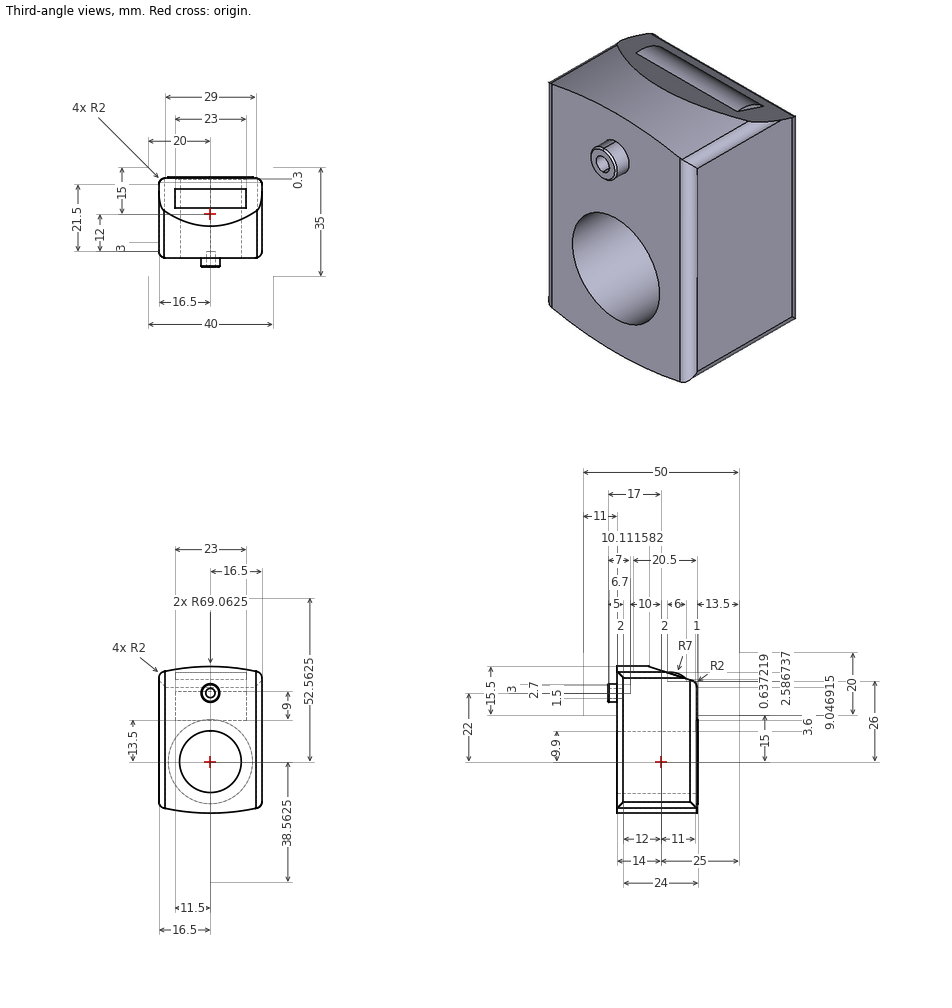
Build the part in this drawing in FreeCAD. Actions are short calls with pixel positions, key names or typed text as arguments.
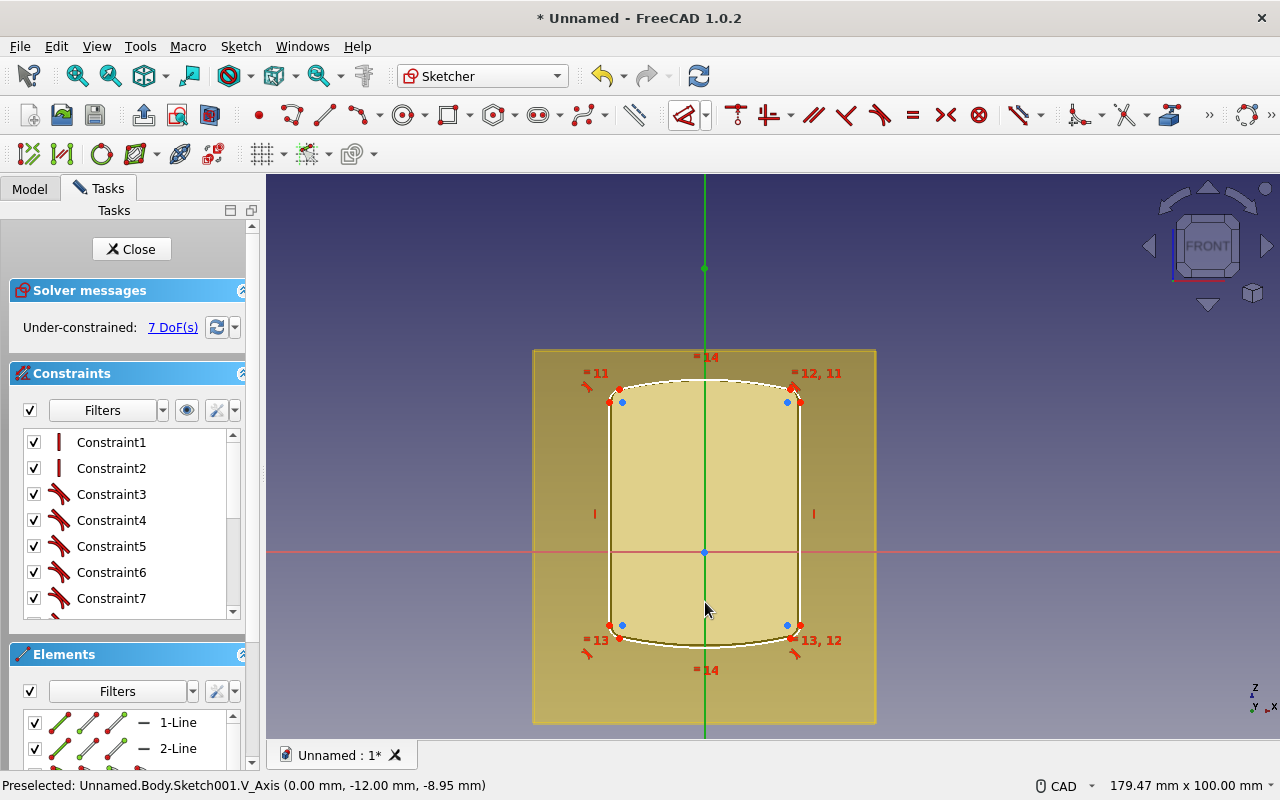
click(736, 116)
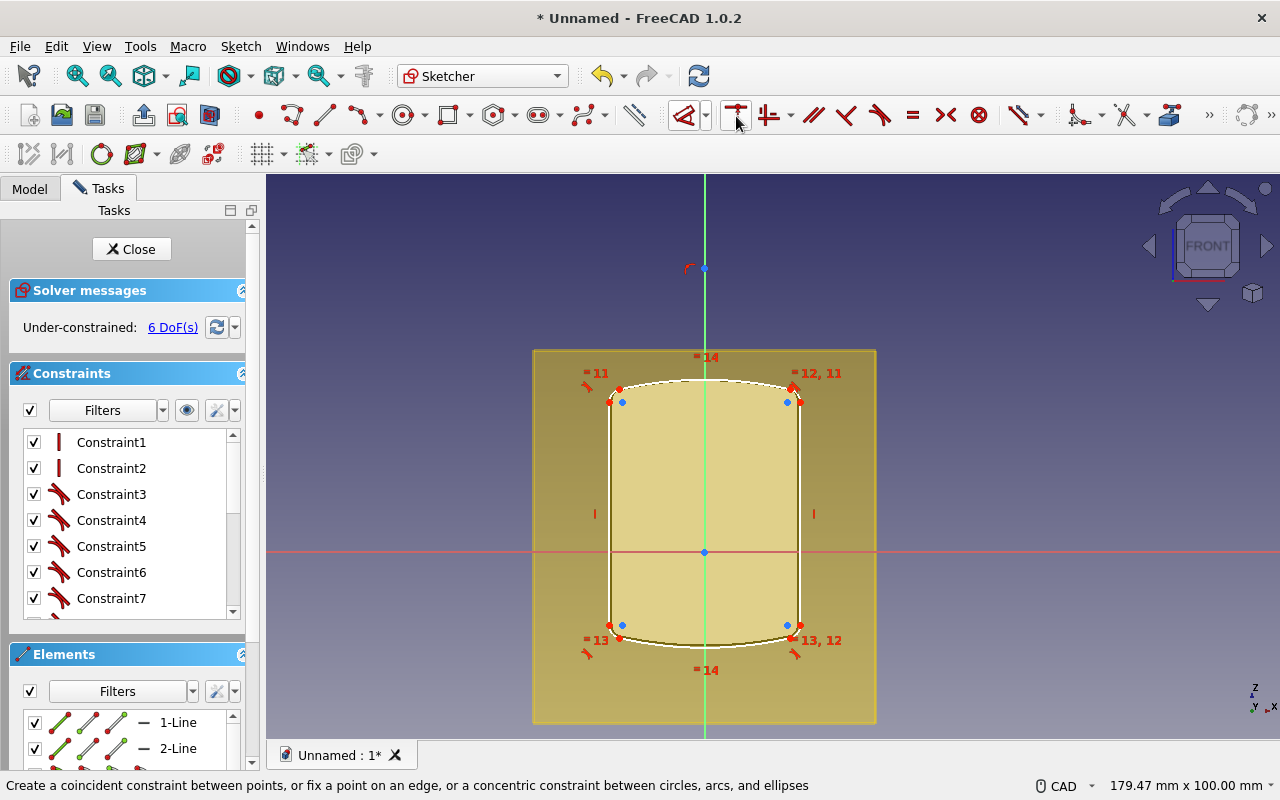
scroll(612, 394, up, 7)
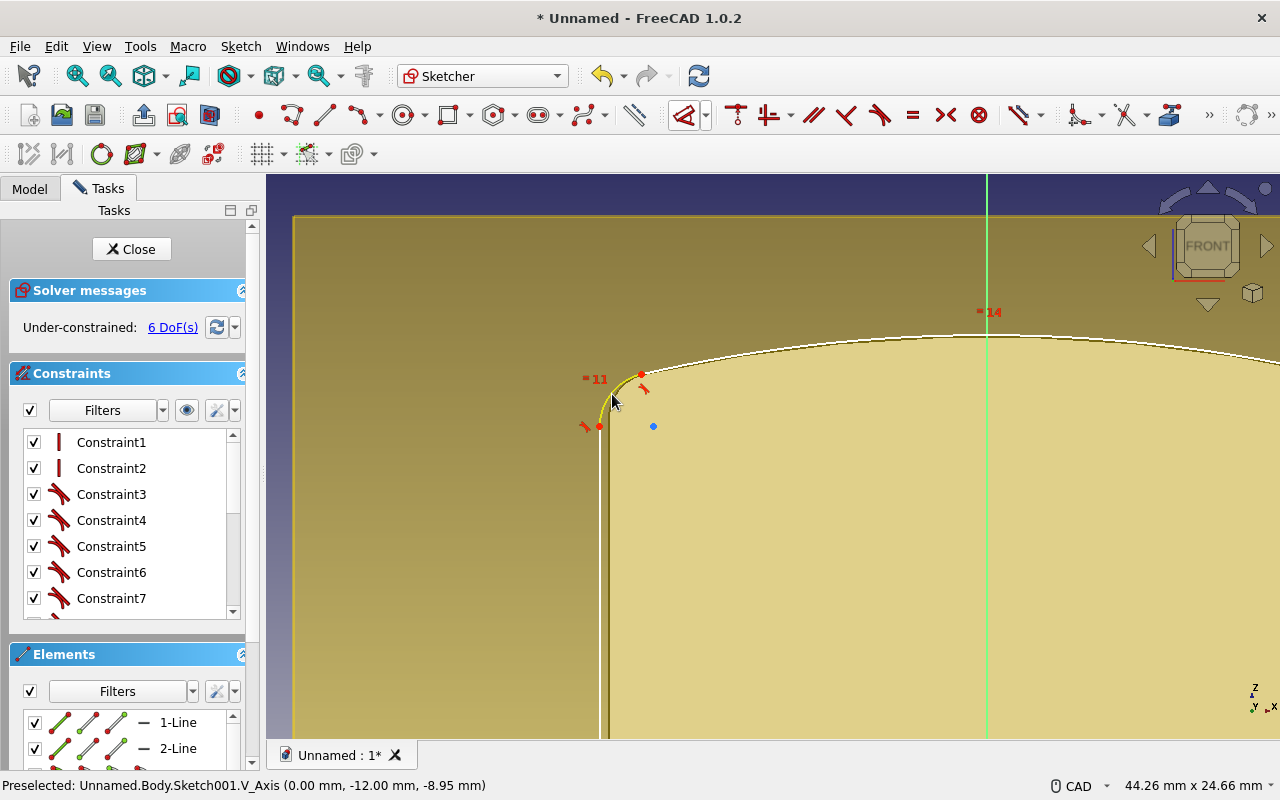
click(612, 393)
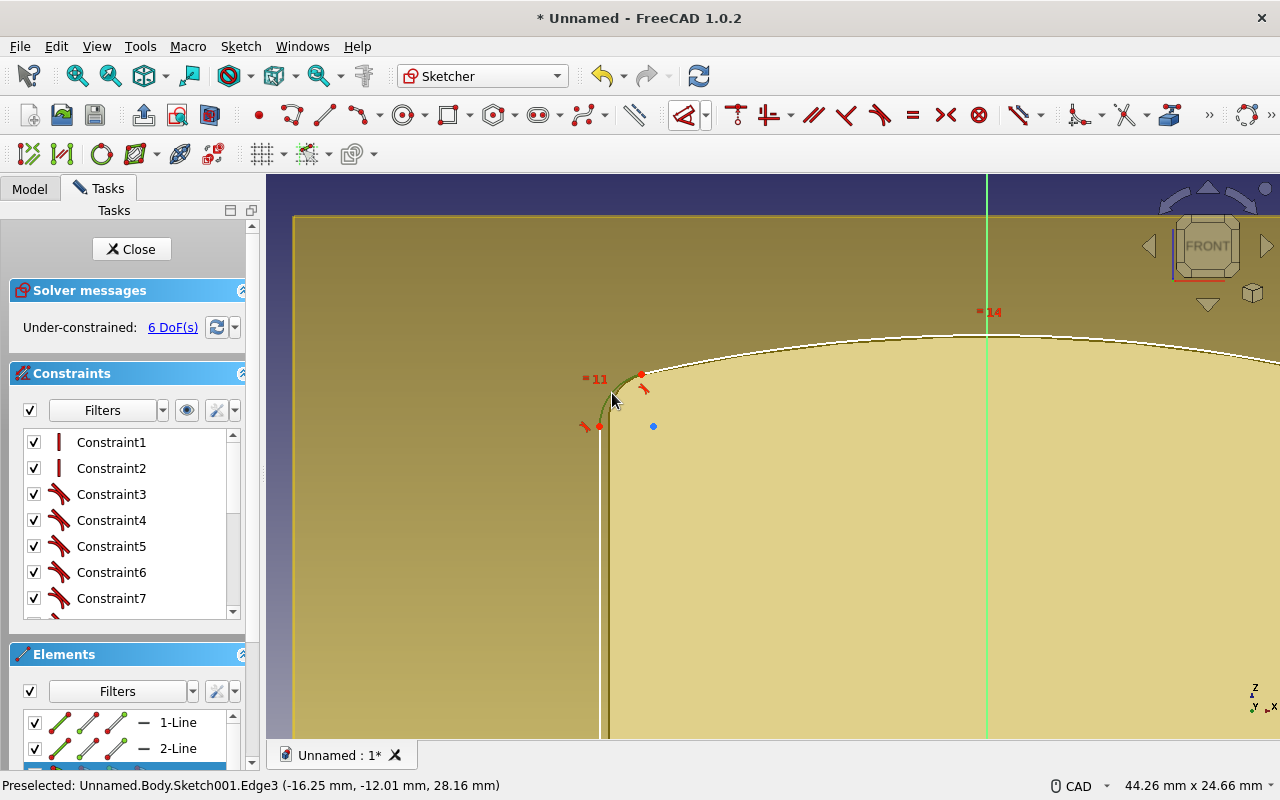
key(k)
key(r)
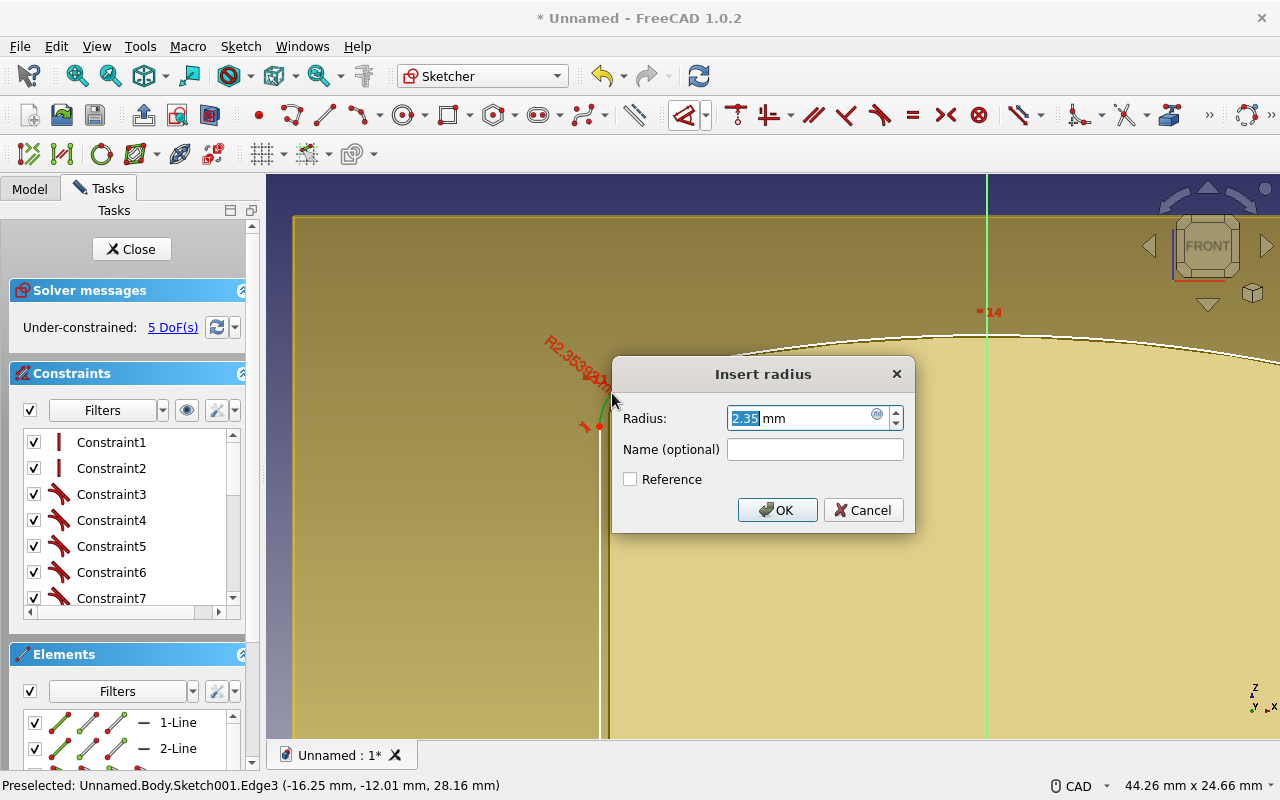
text(2)
key(Return)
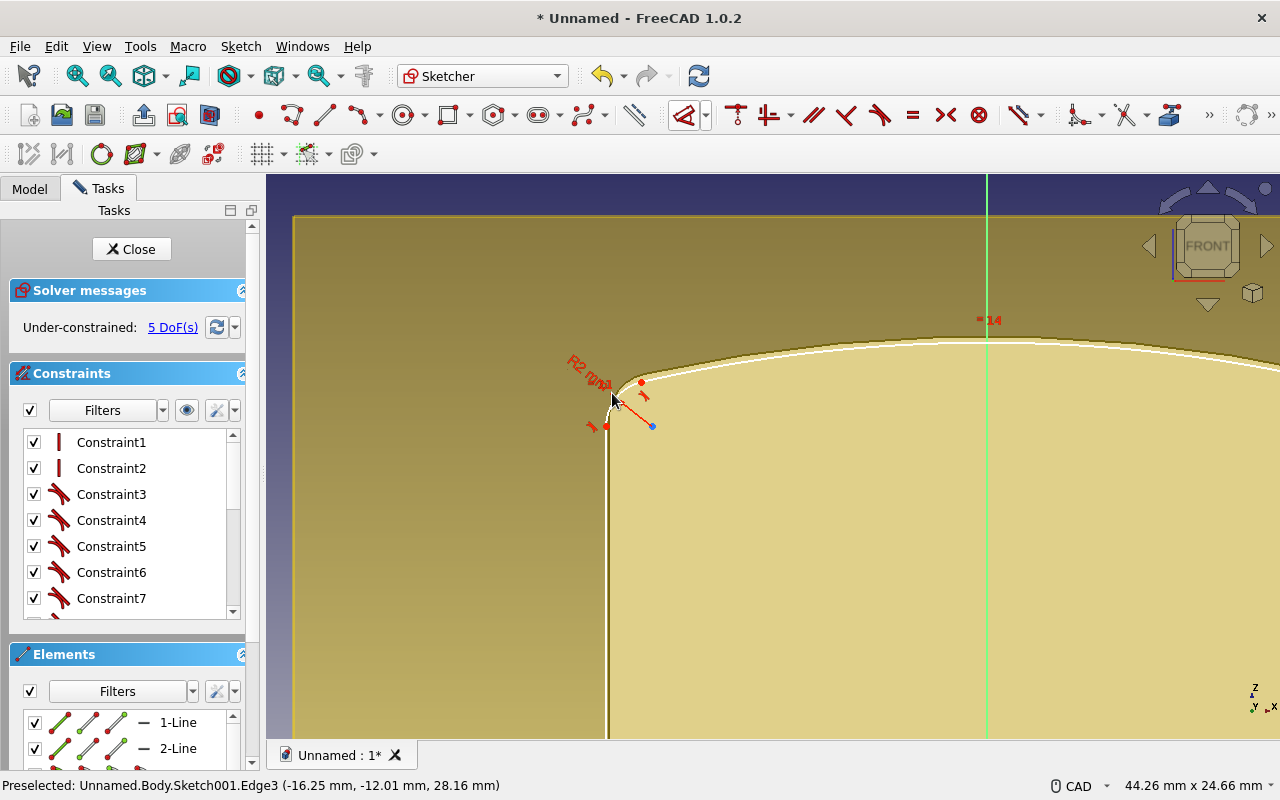
click(848, 349)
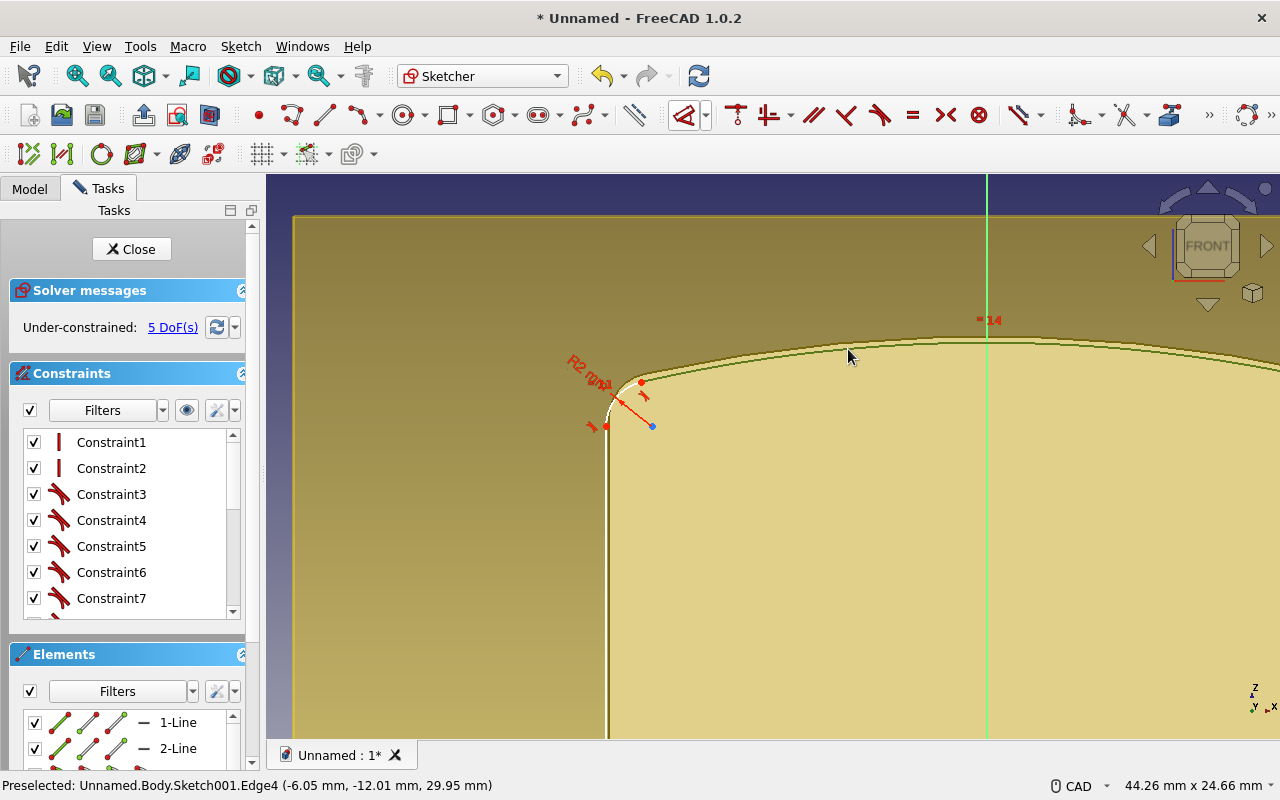
click(706, 116)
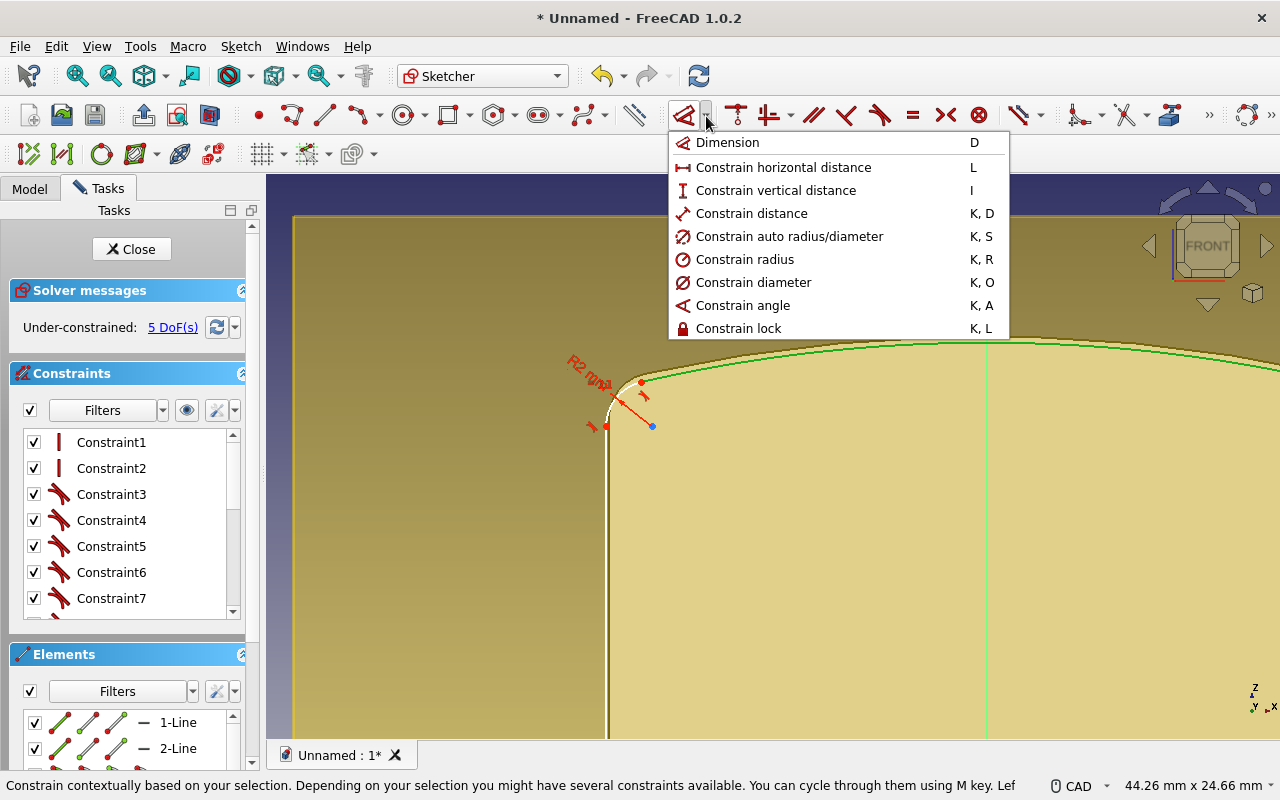
click(839, 260)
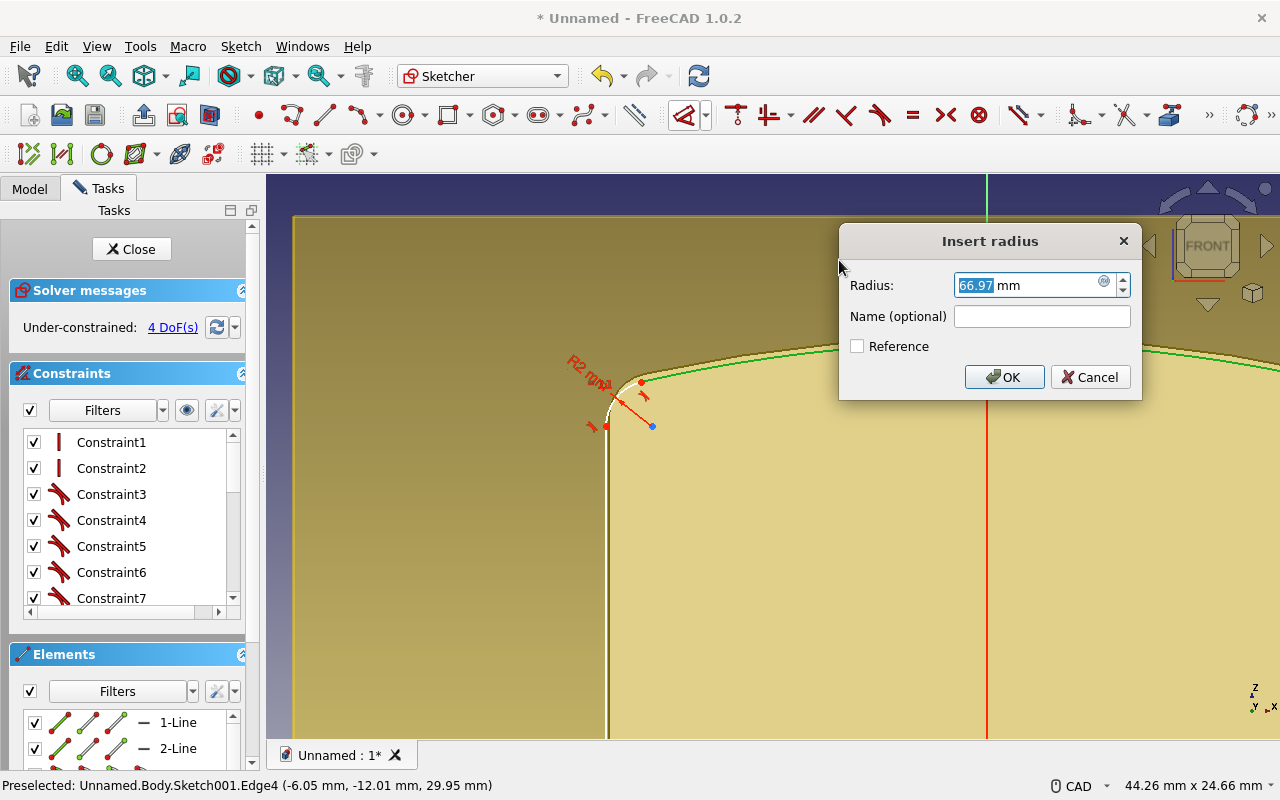
text(69.0625)
key(Return)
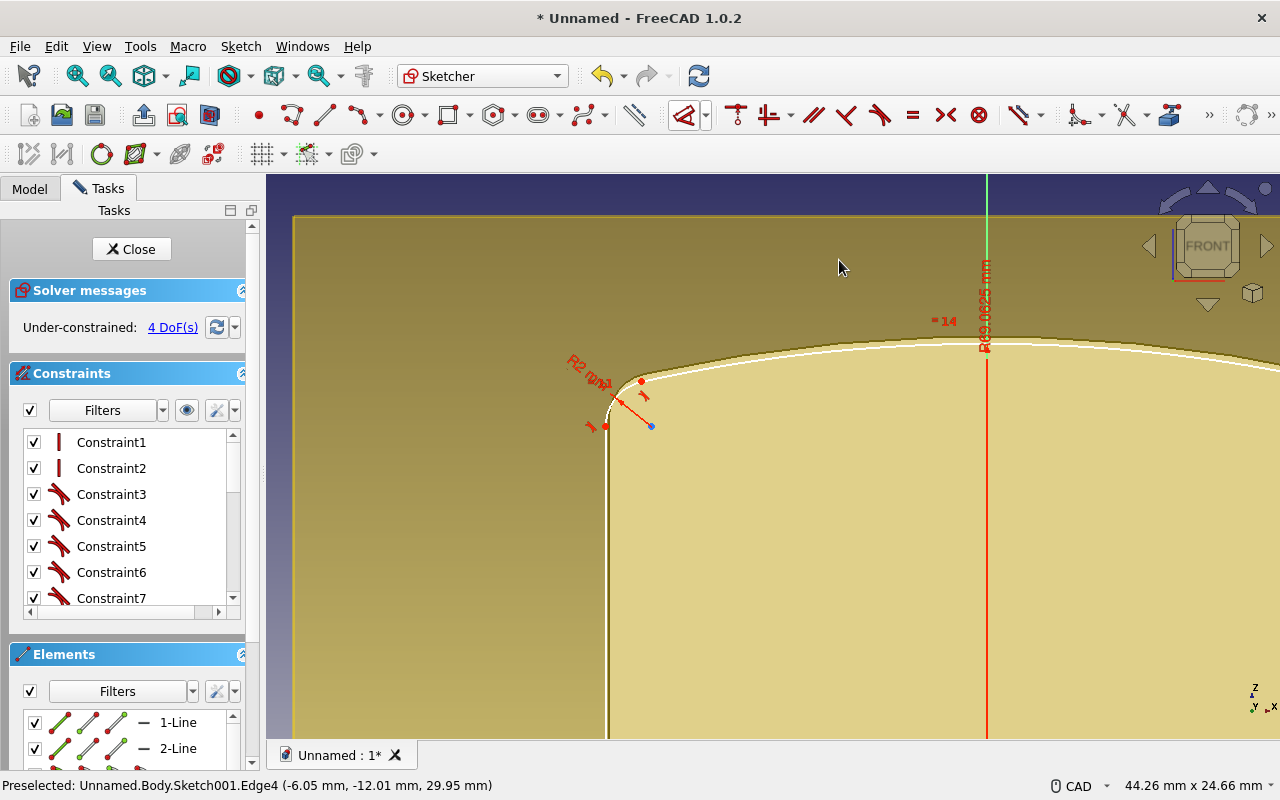
scroll(540, 213, down, 5)